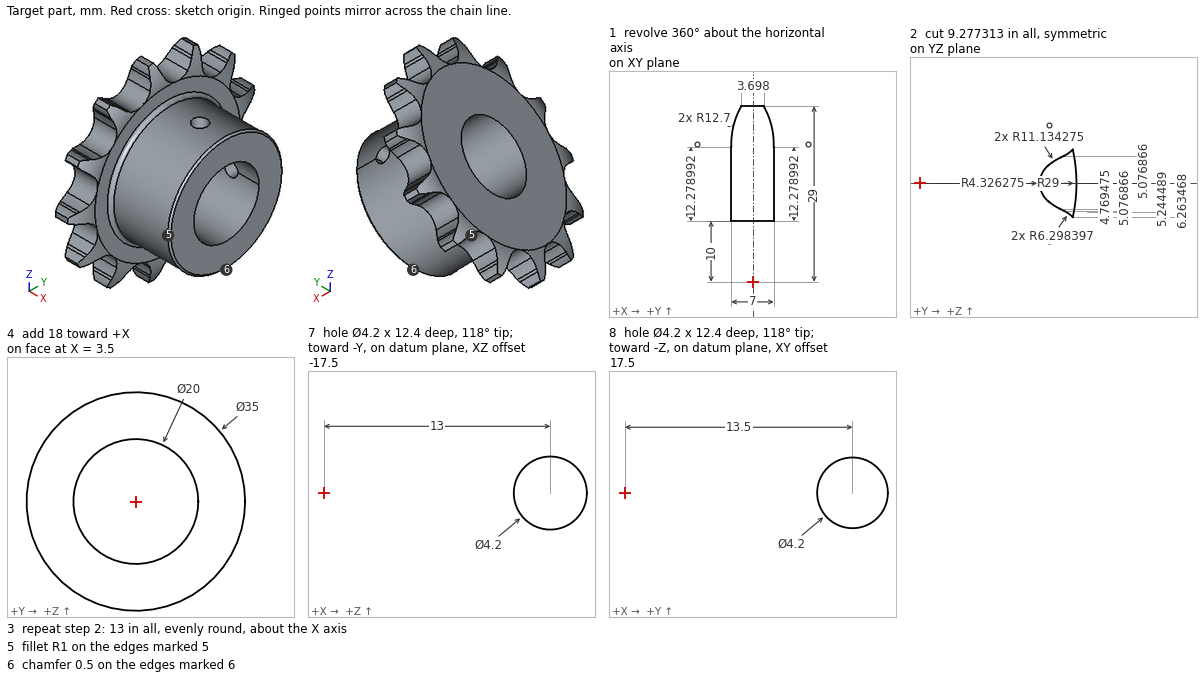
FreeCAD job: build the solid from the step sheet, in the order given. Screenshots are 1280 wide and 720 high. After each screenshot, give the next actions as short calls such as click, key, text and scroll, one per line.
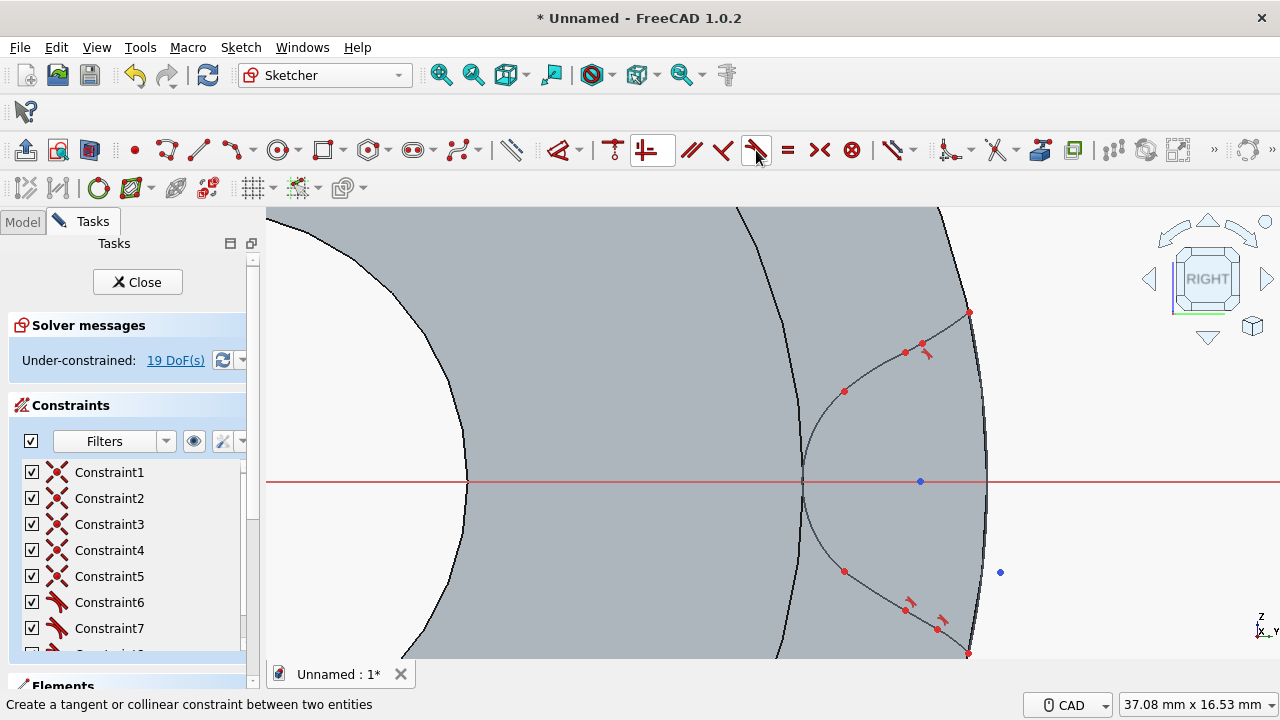
scroll(914, 348, up, 2)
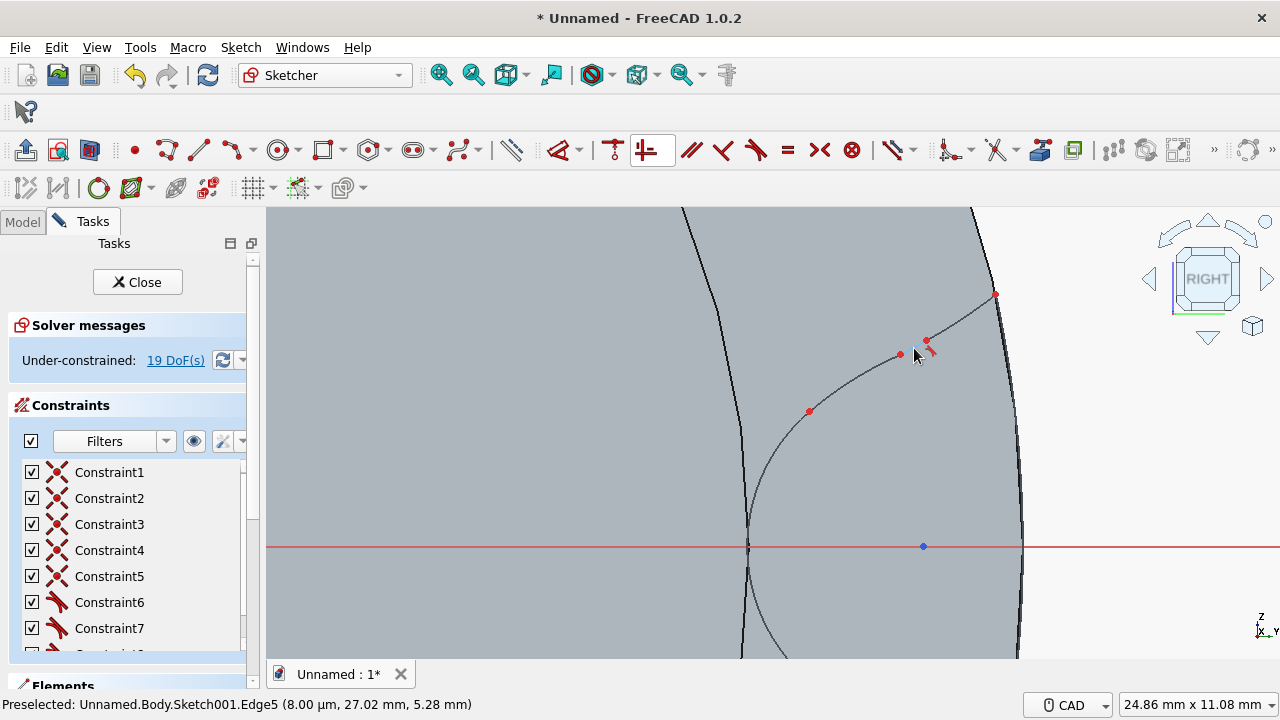
click(914, 348)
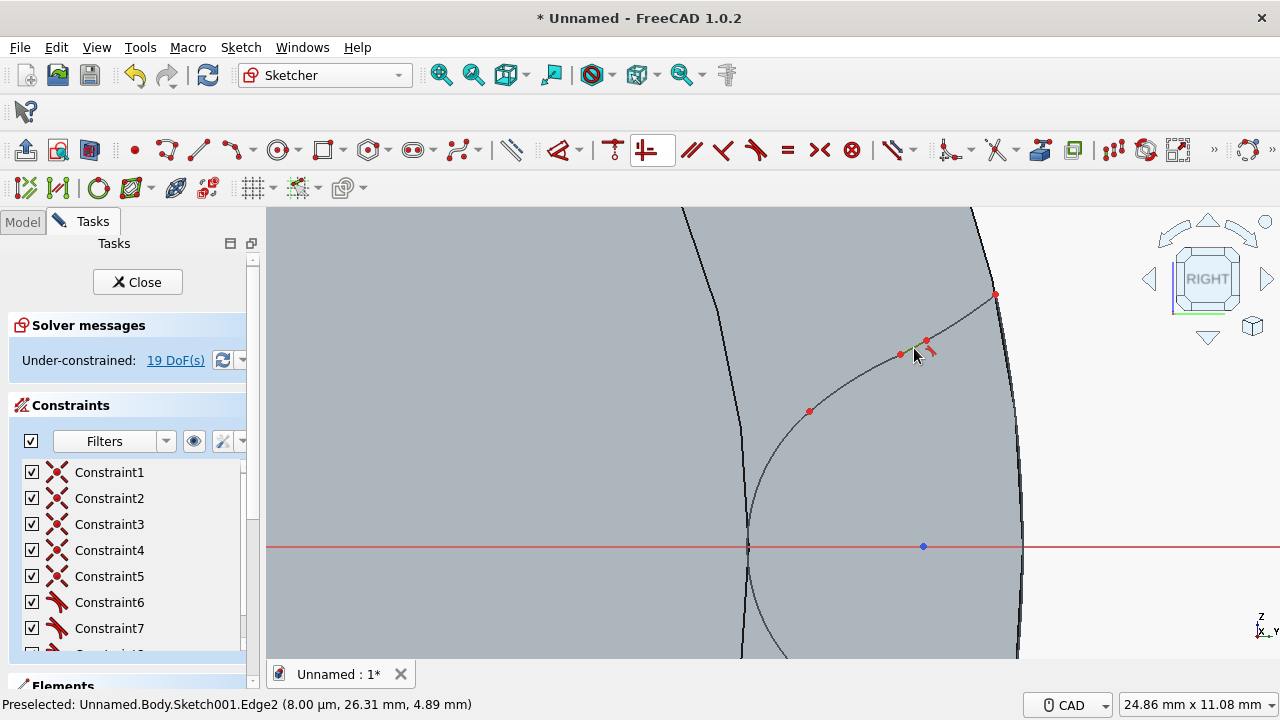
click(872, 369)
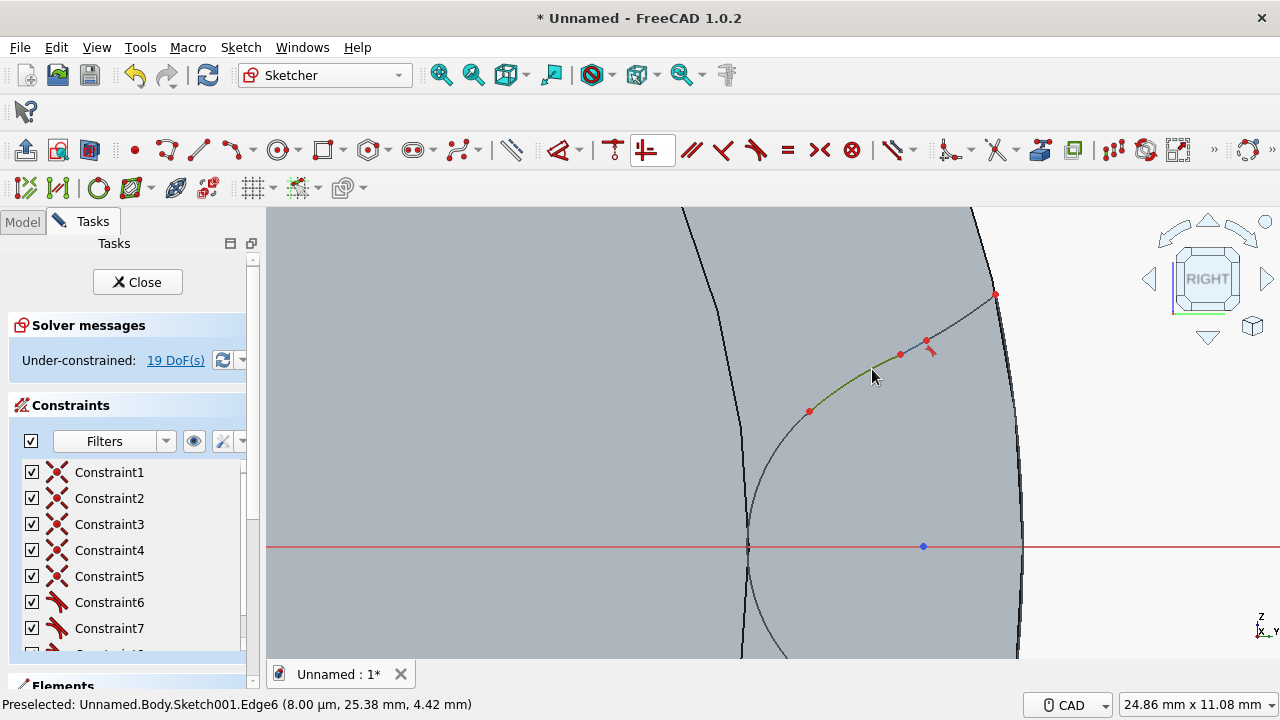
key(t)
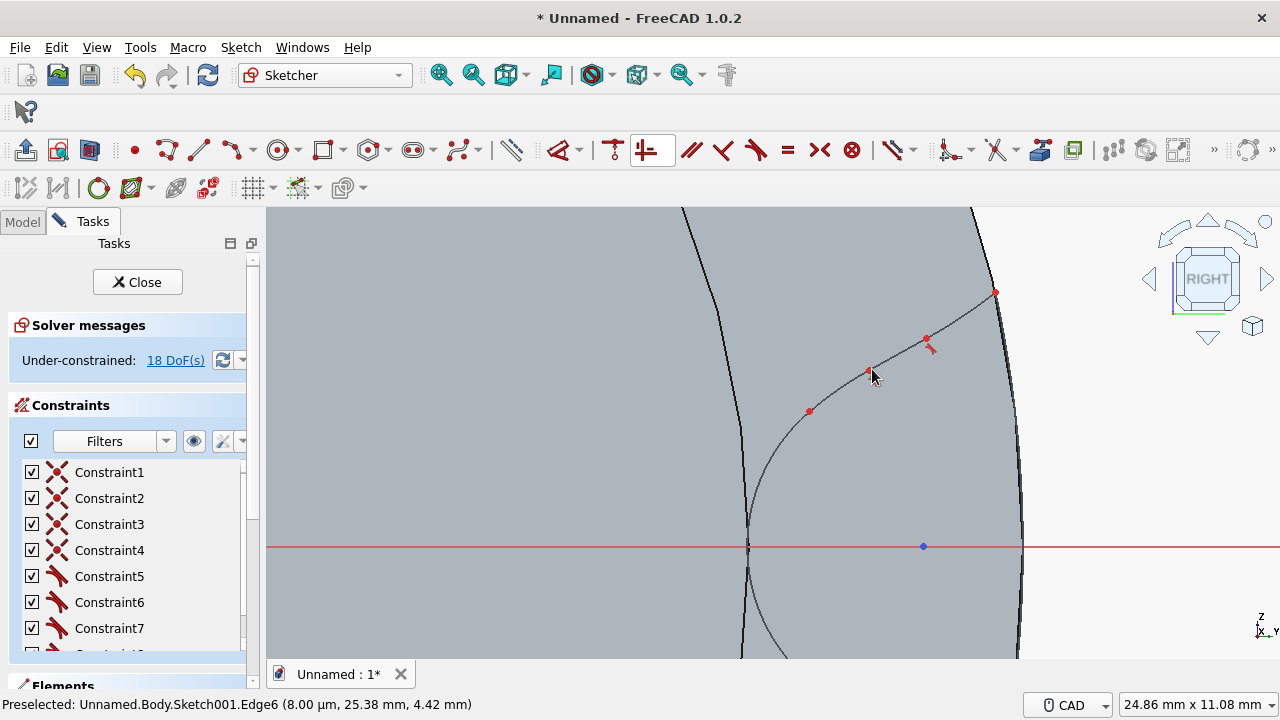
click(850, 381)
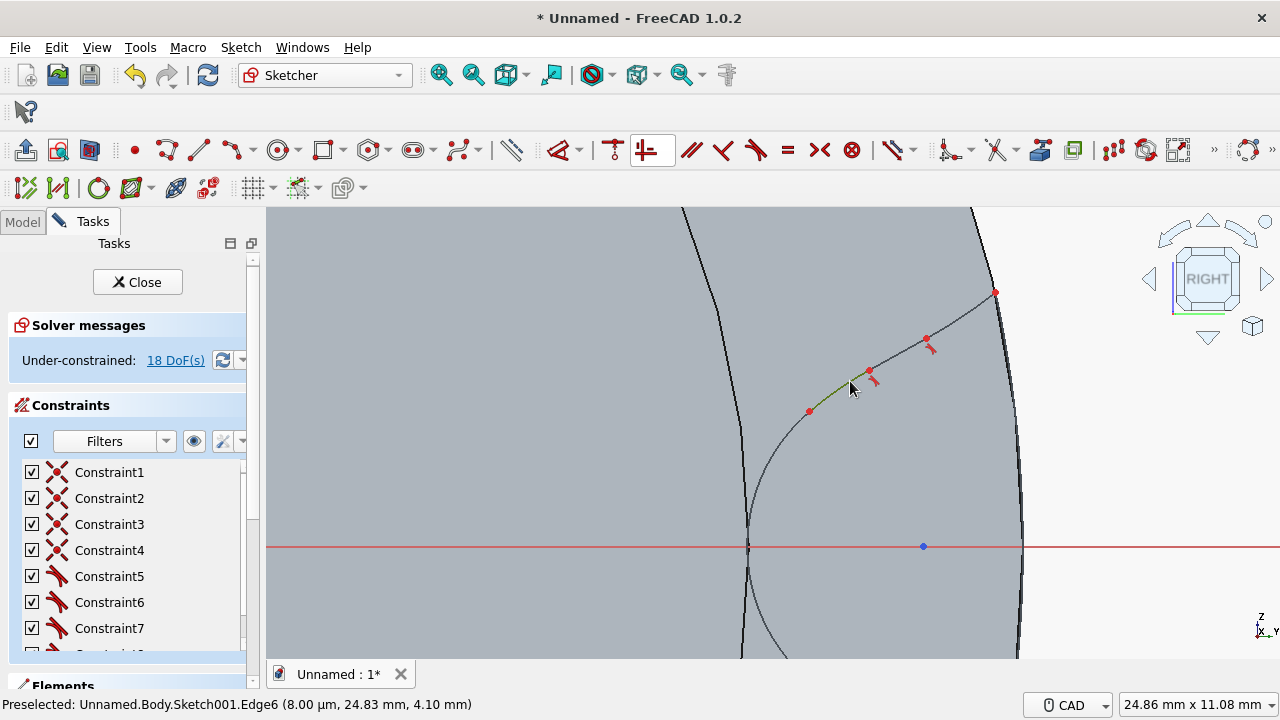
click(758, 487)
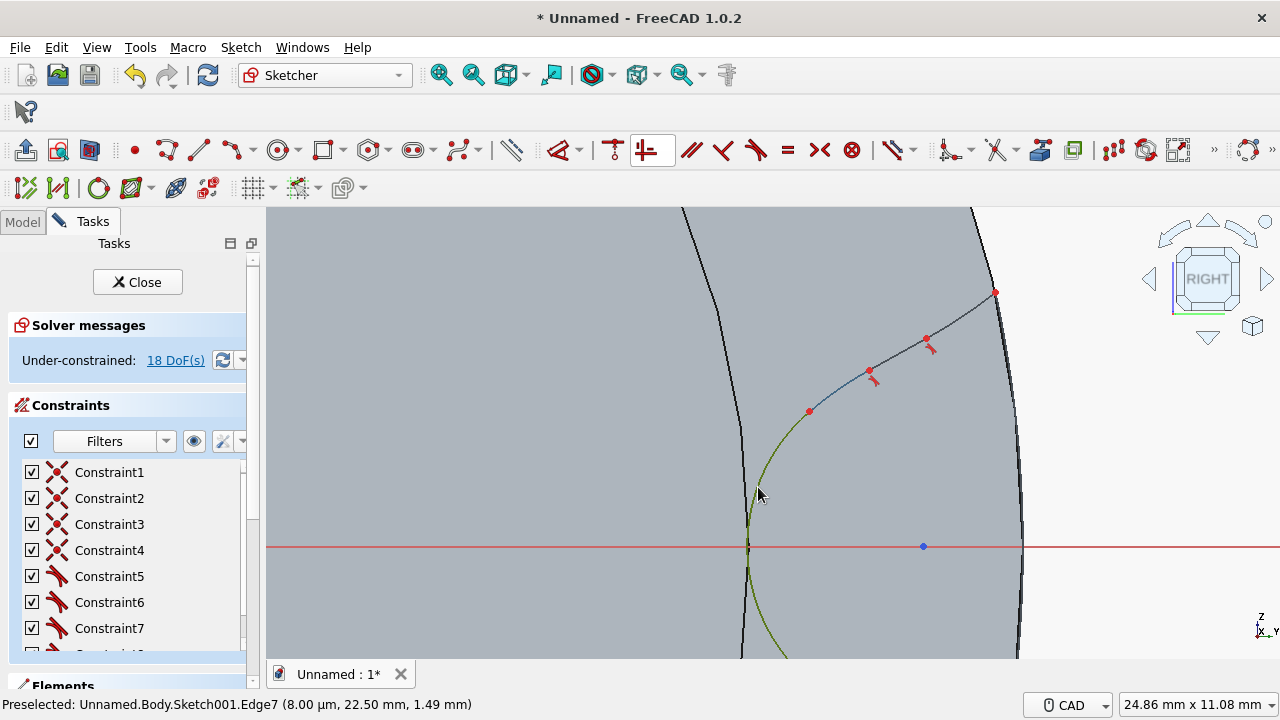
click(756, 150)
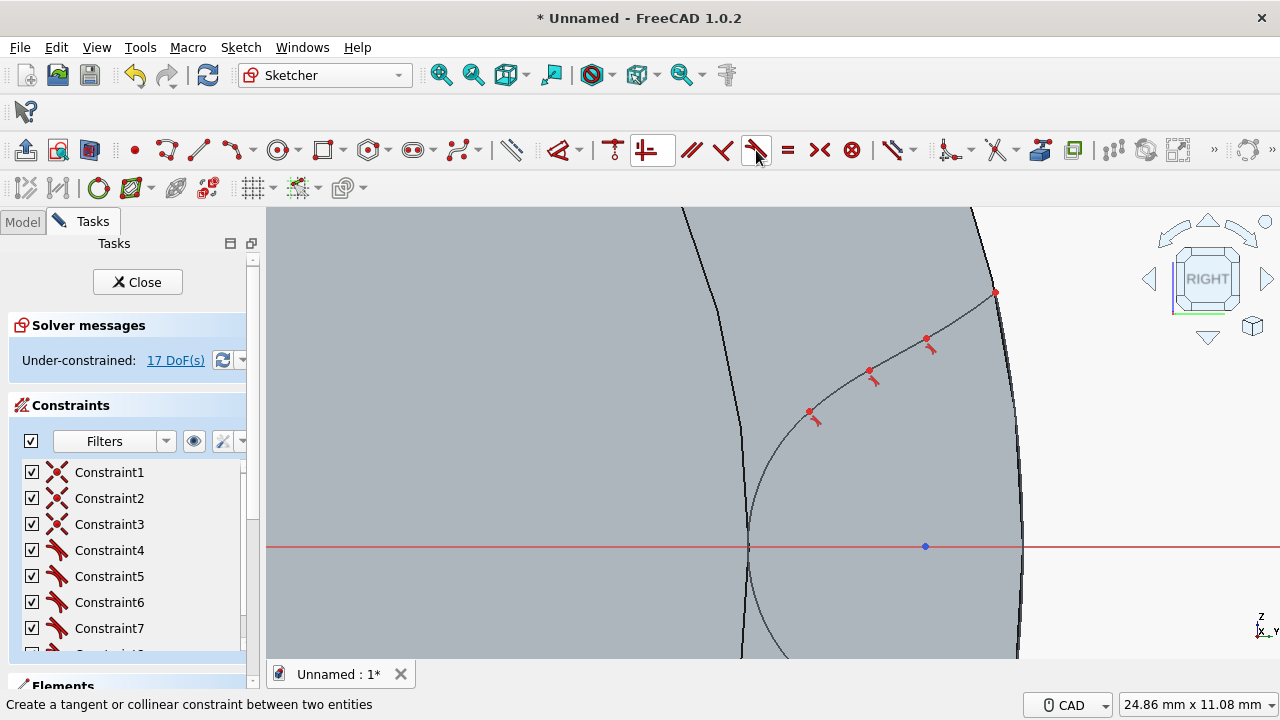
click(758, 487)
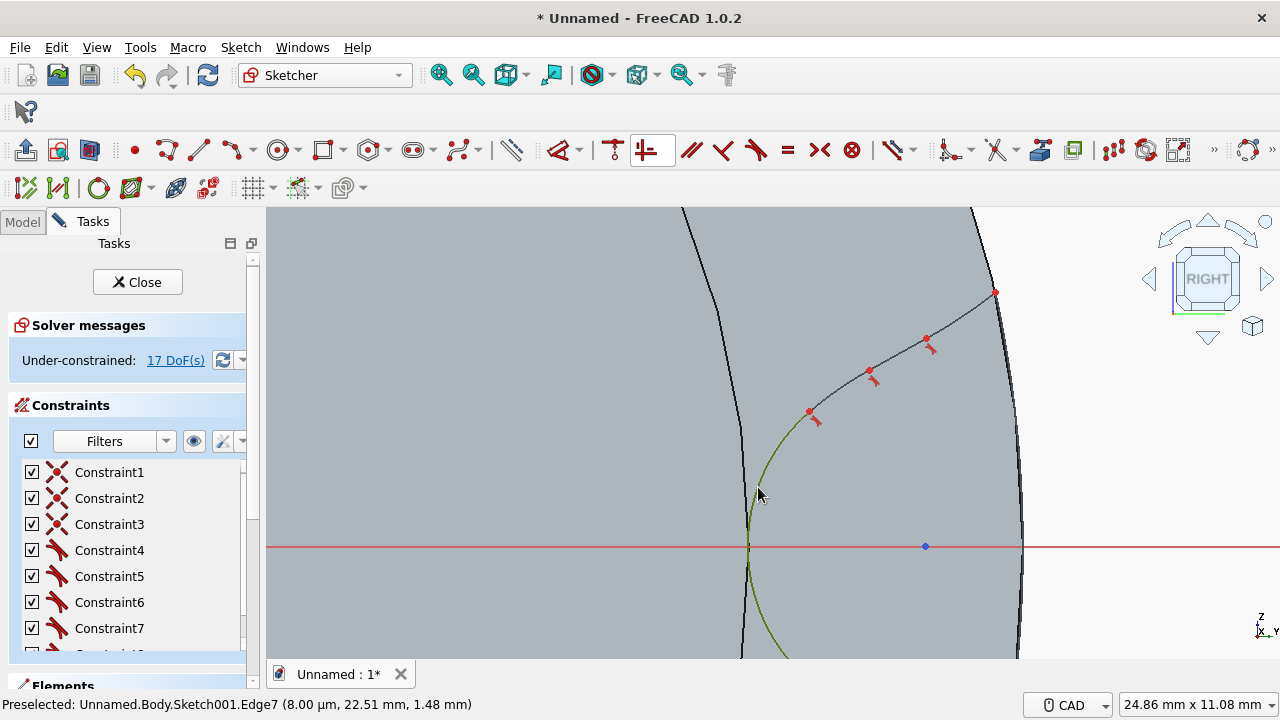
scroll(927, 340, down, 4)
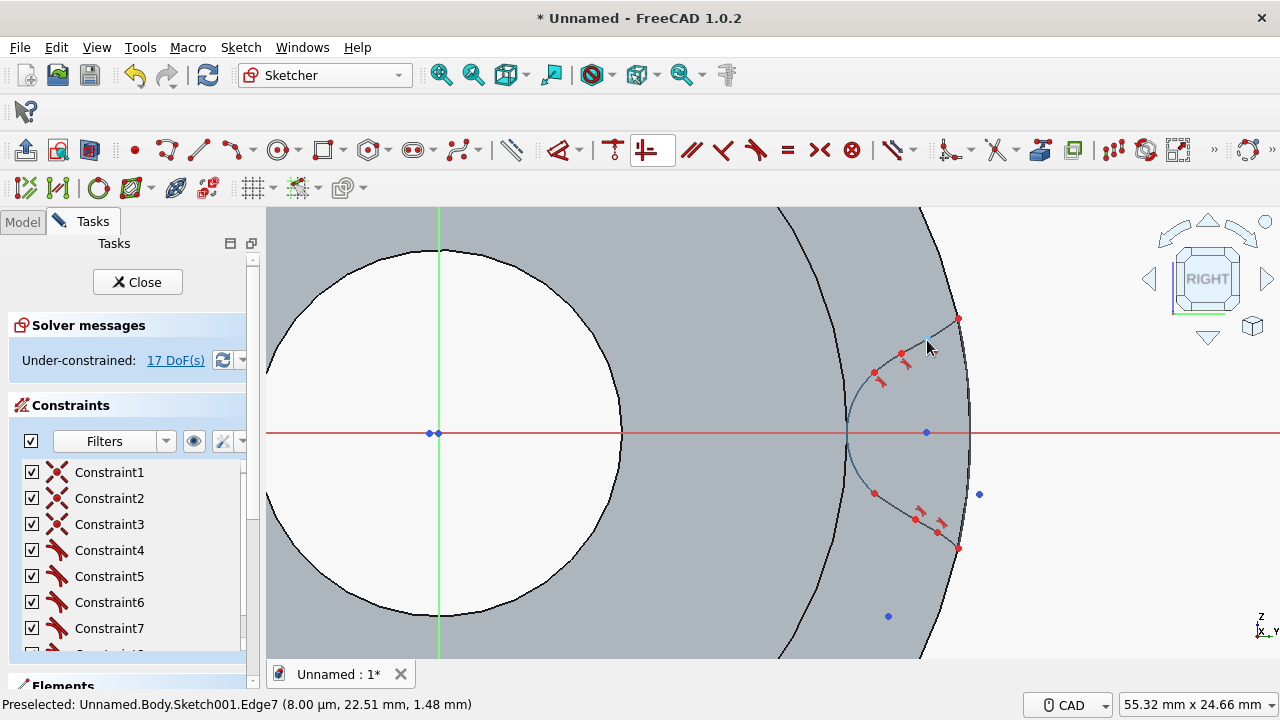
click(887, 502)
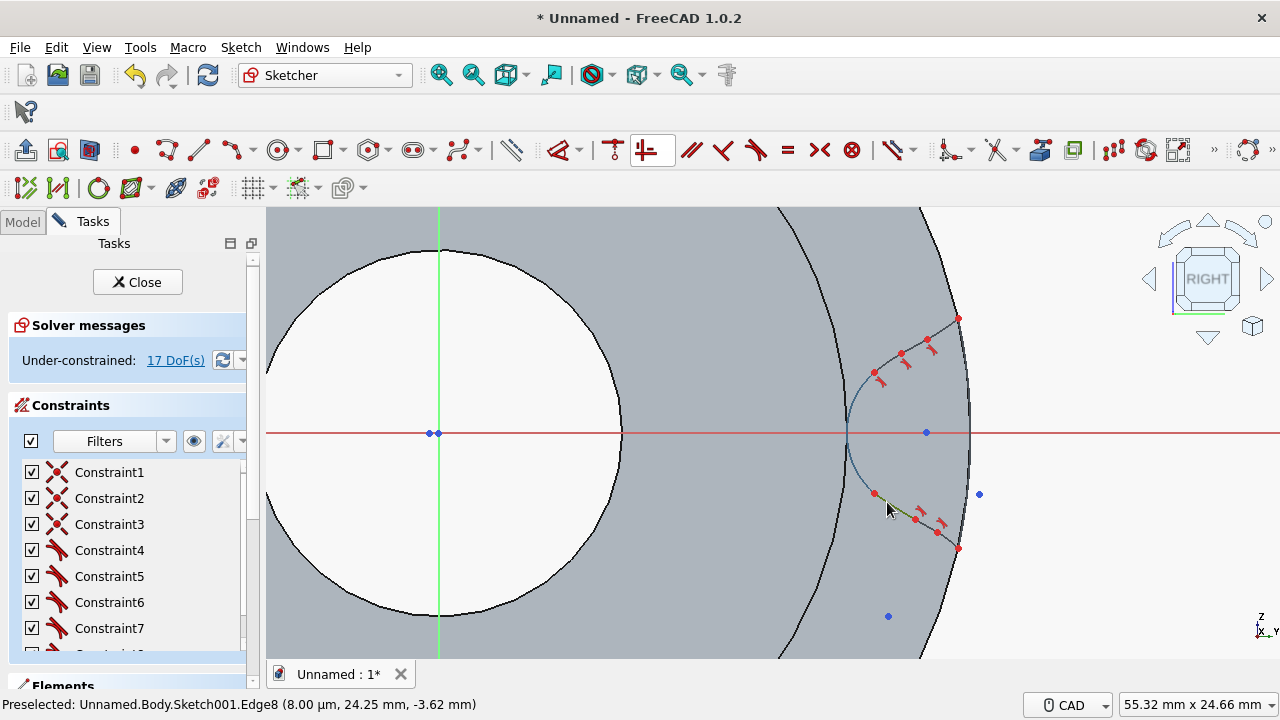
click(756, 150)